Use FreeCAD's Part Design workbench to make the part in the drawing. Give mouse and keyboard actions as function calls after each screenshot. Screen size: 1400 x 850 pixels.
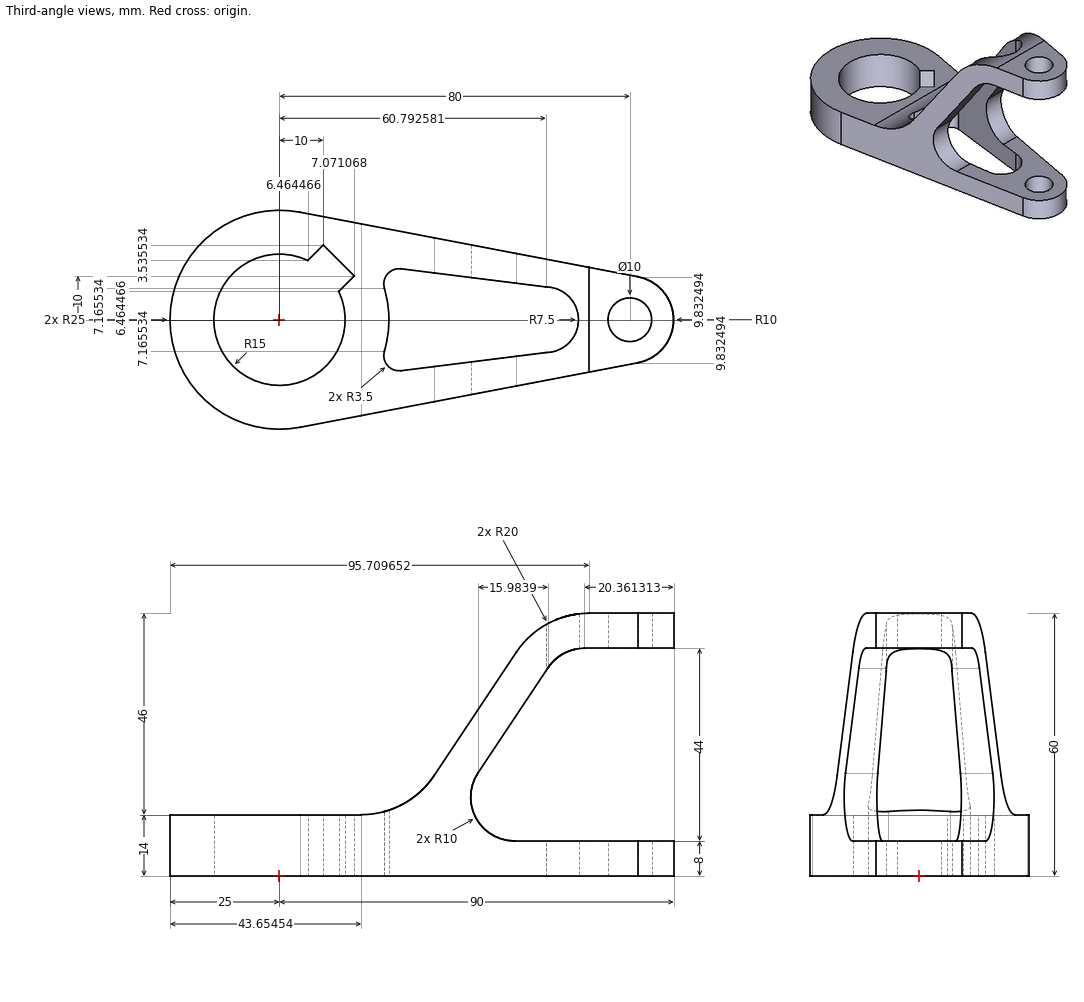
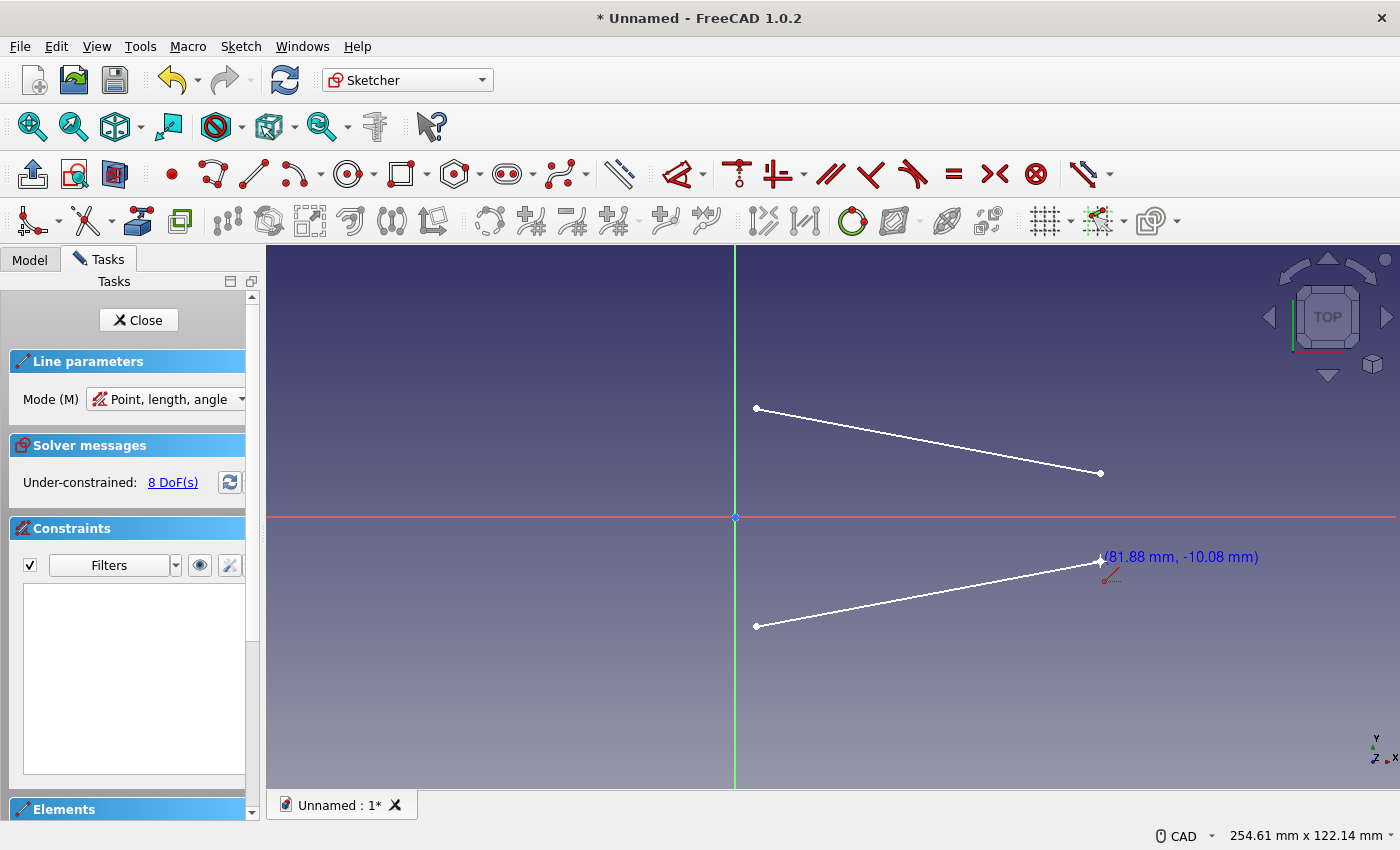
click(320, 174)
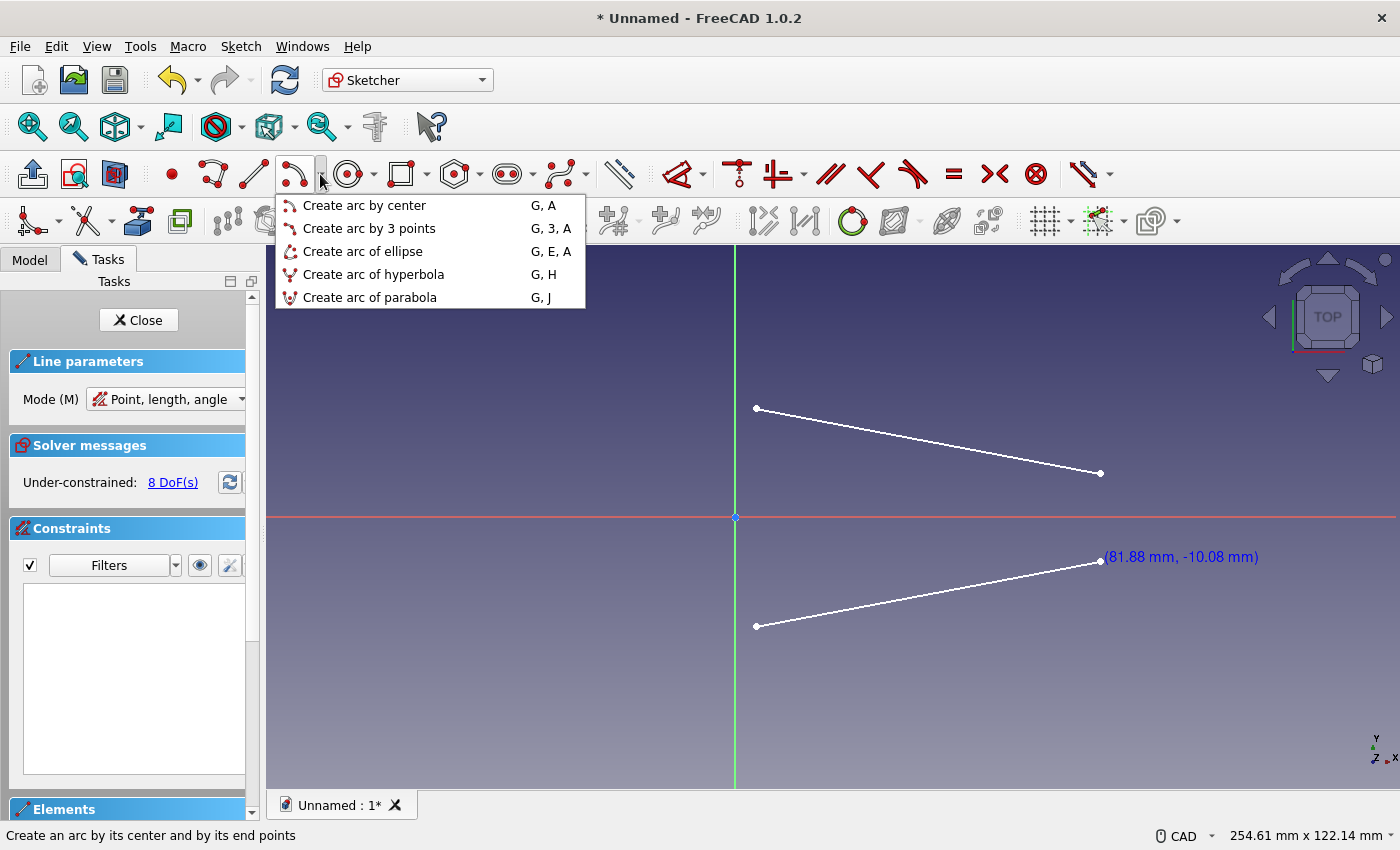
click(430, 228)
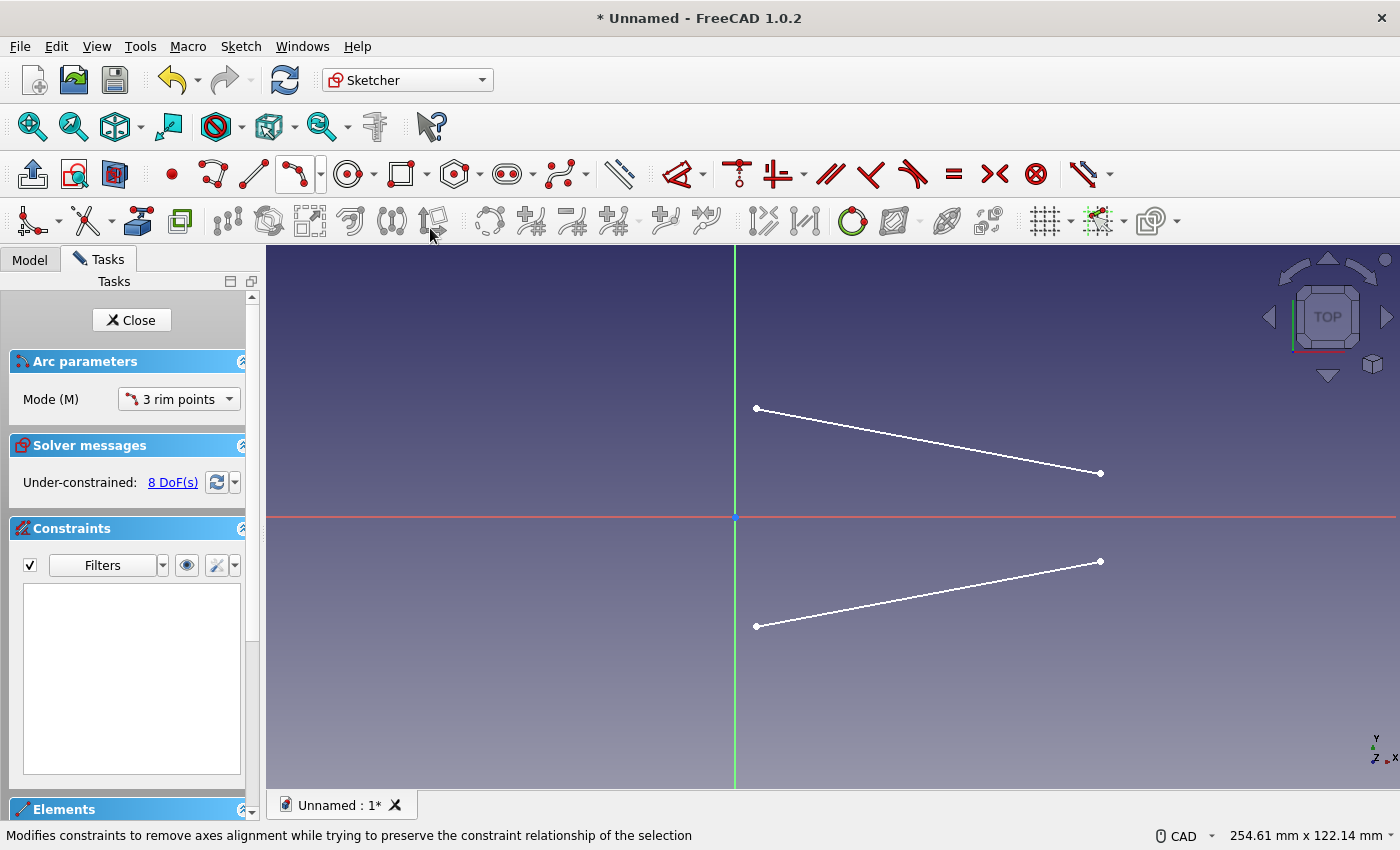
click(756, 409)
click(756, 627)
click(631, 479)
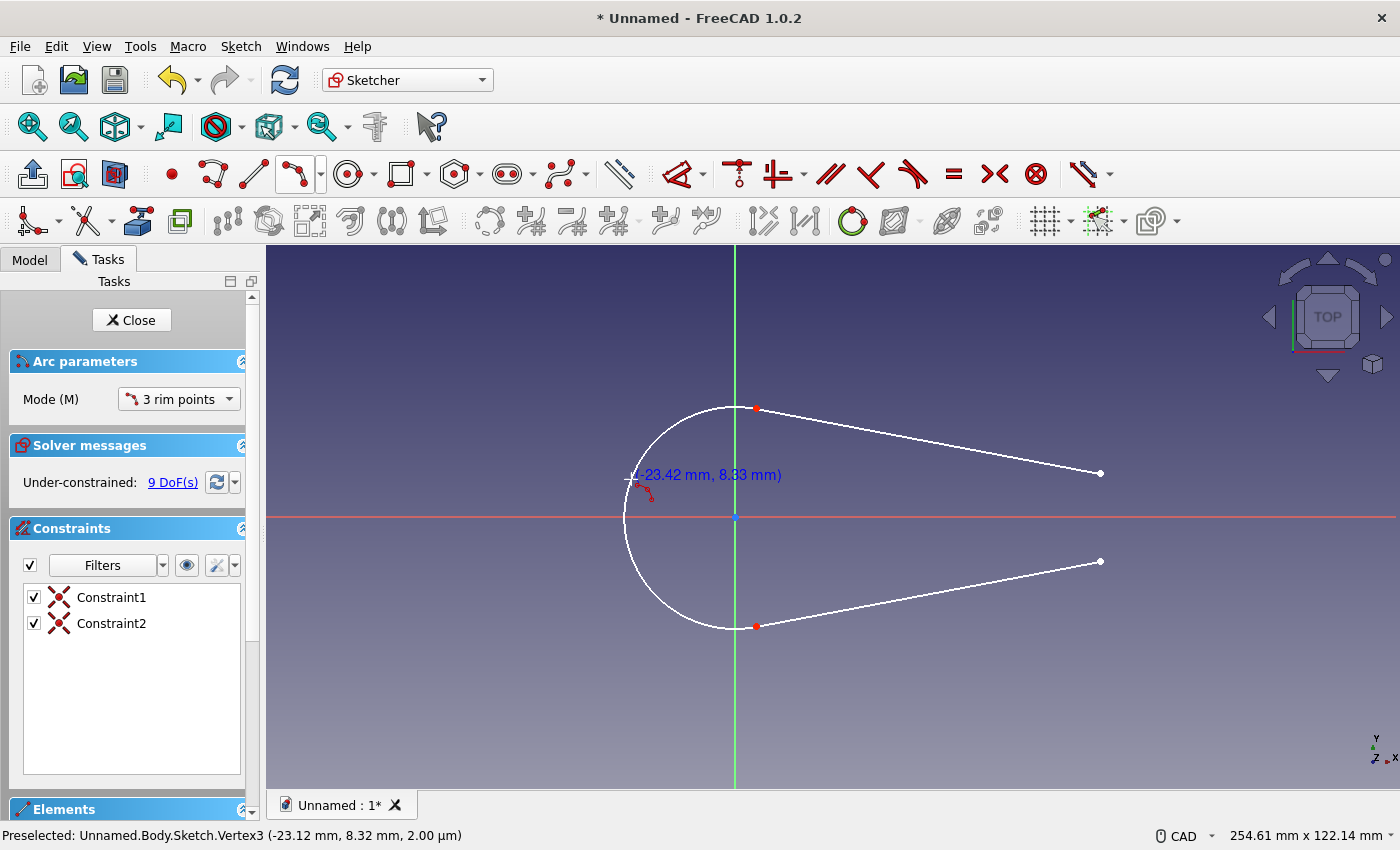
click(1100, 562)
click(1100, 474)
click(1129, 541)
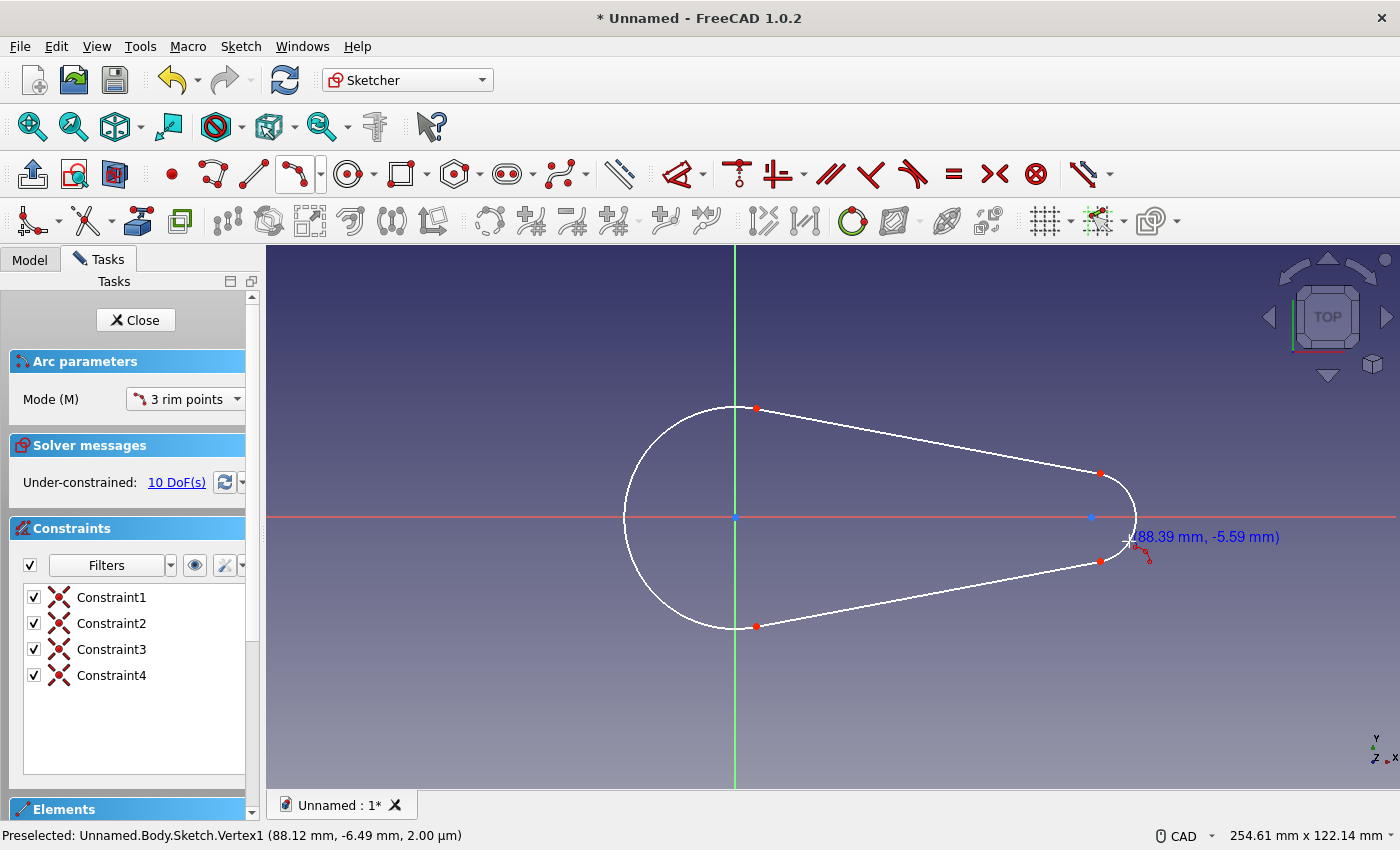
click(254, 174)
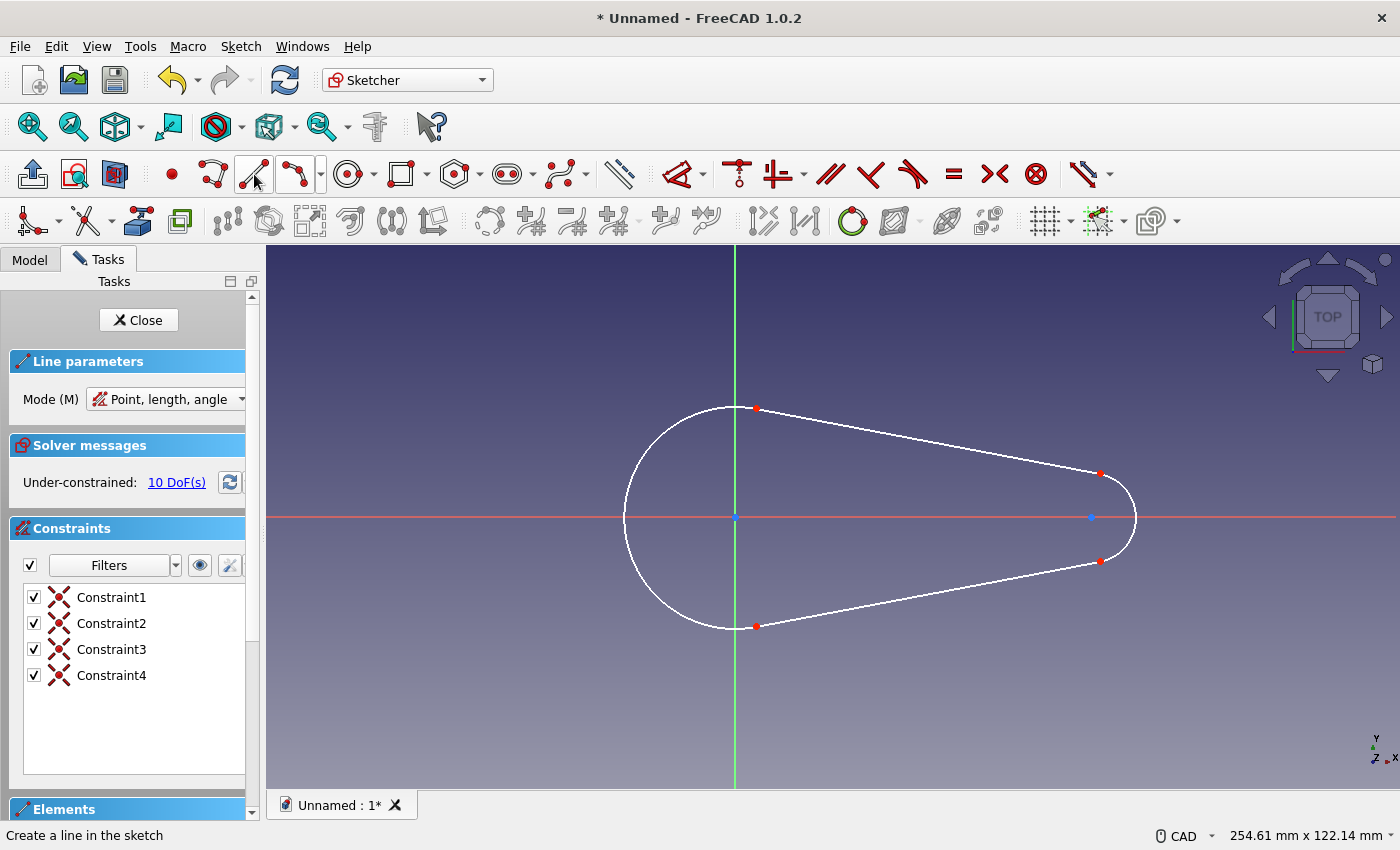
click(859, 465)
click(1006, 484)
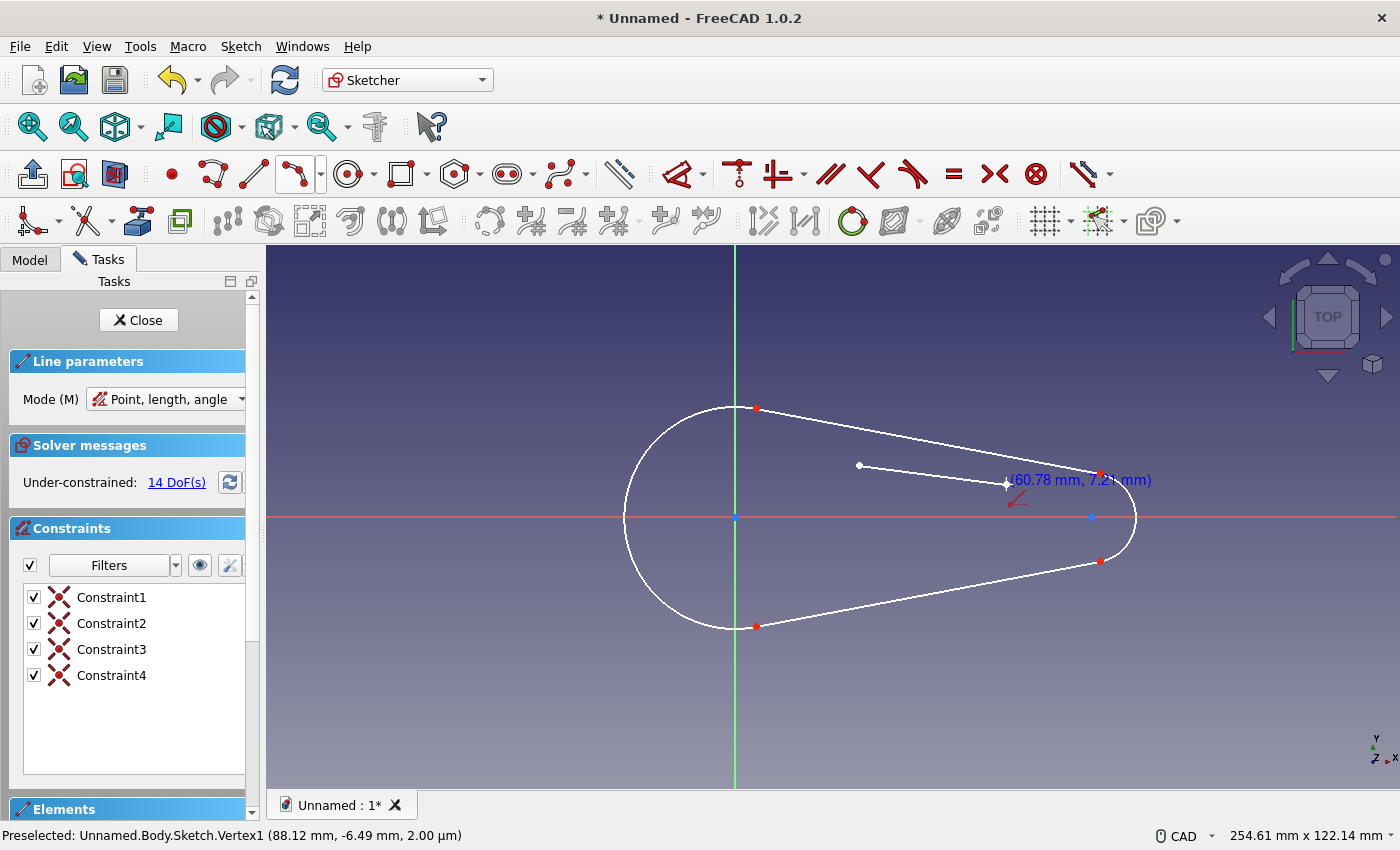
click(1006, 550)
click(859, 569)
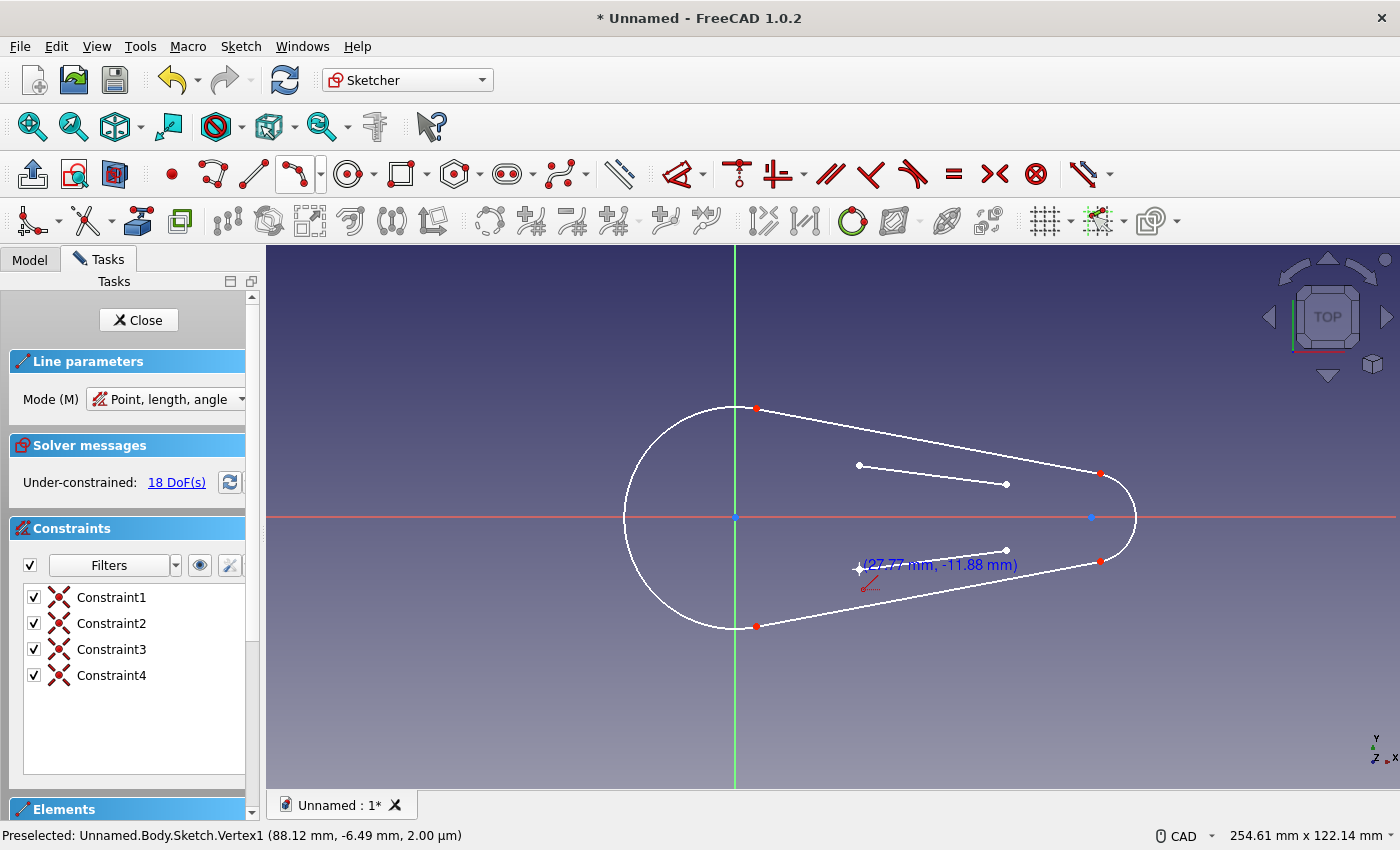
key(g)
key(3)
key(a)